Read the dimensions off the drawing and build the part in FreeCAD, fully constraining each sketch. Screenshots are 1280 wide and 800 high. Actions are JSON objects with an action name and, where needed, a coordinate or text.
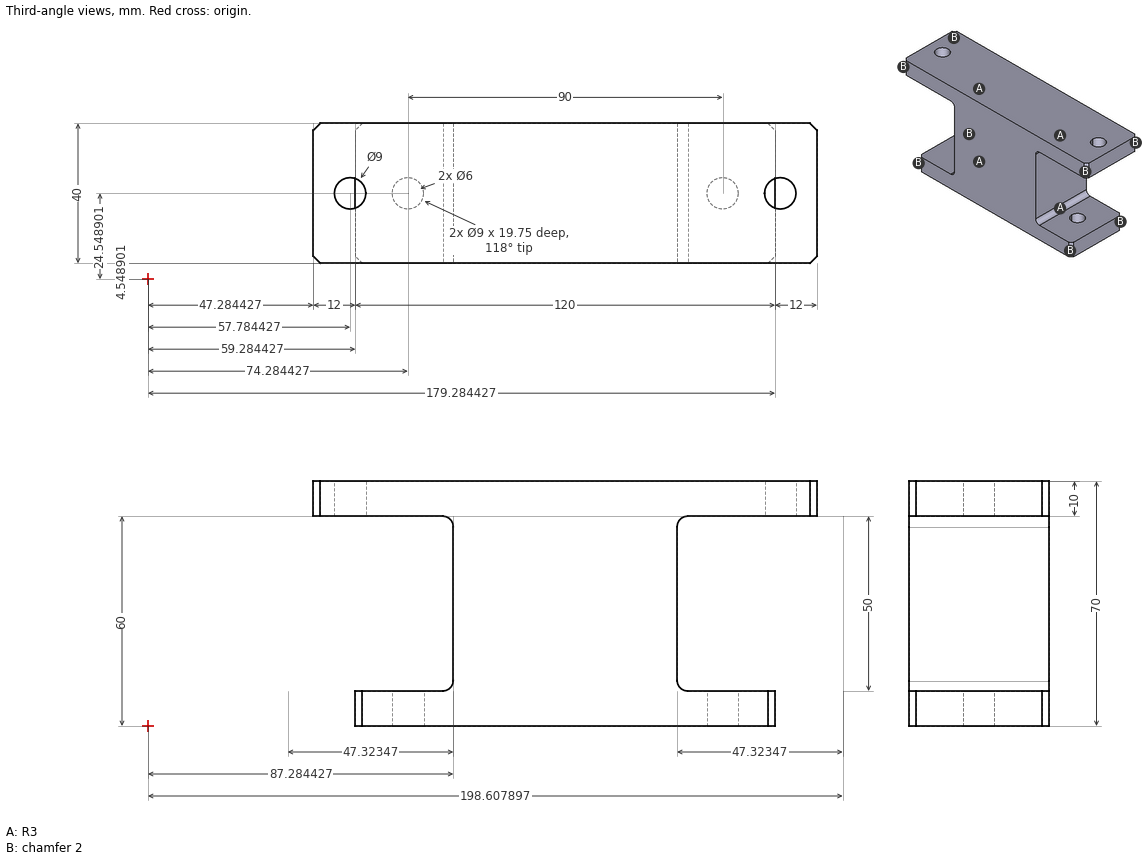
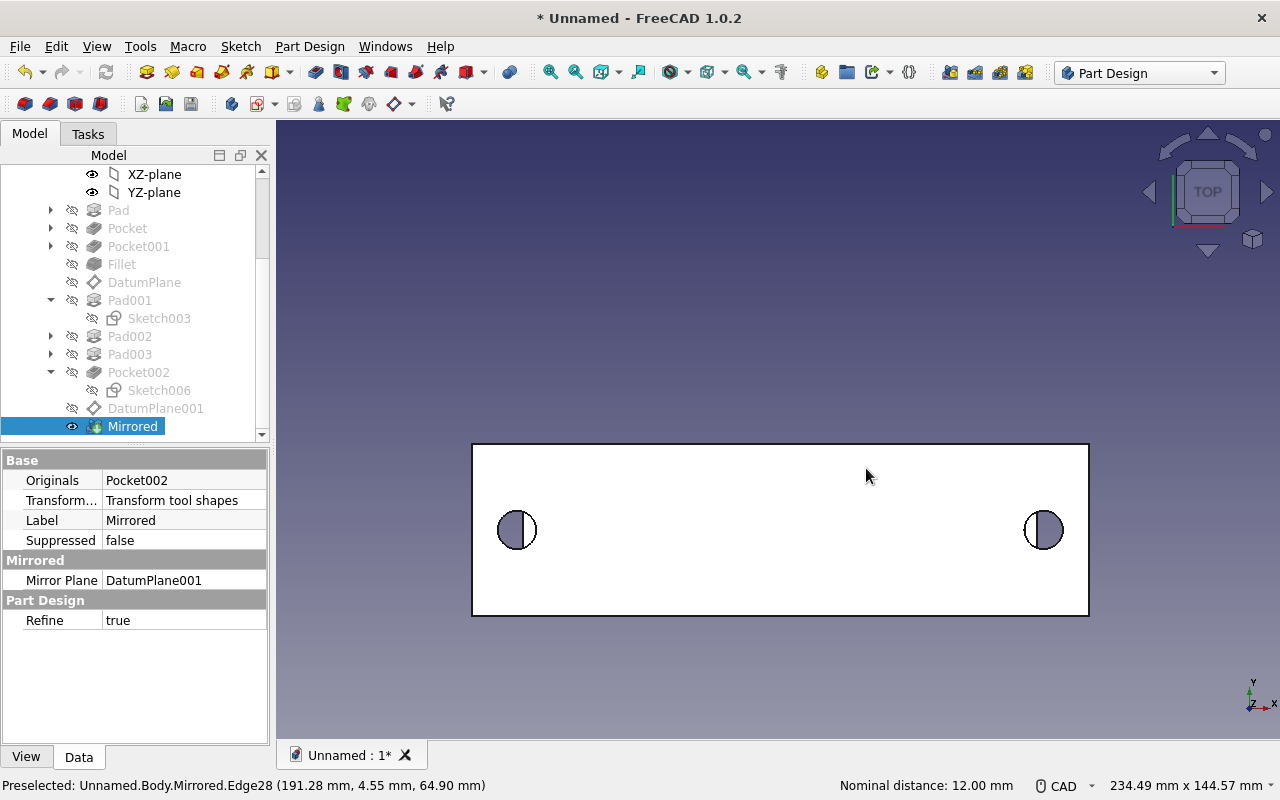
{"action": "key", "text": "0"}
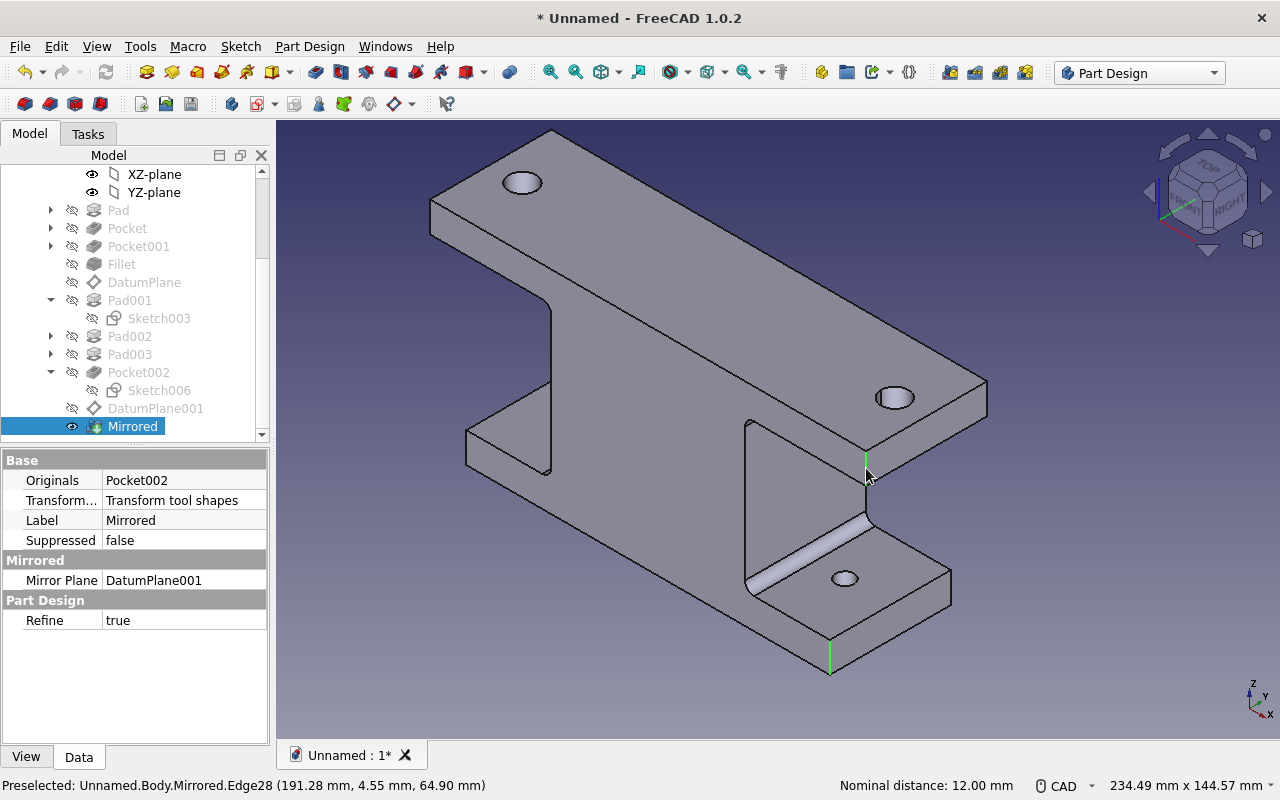
{"action": "key", "text": "1"}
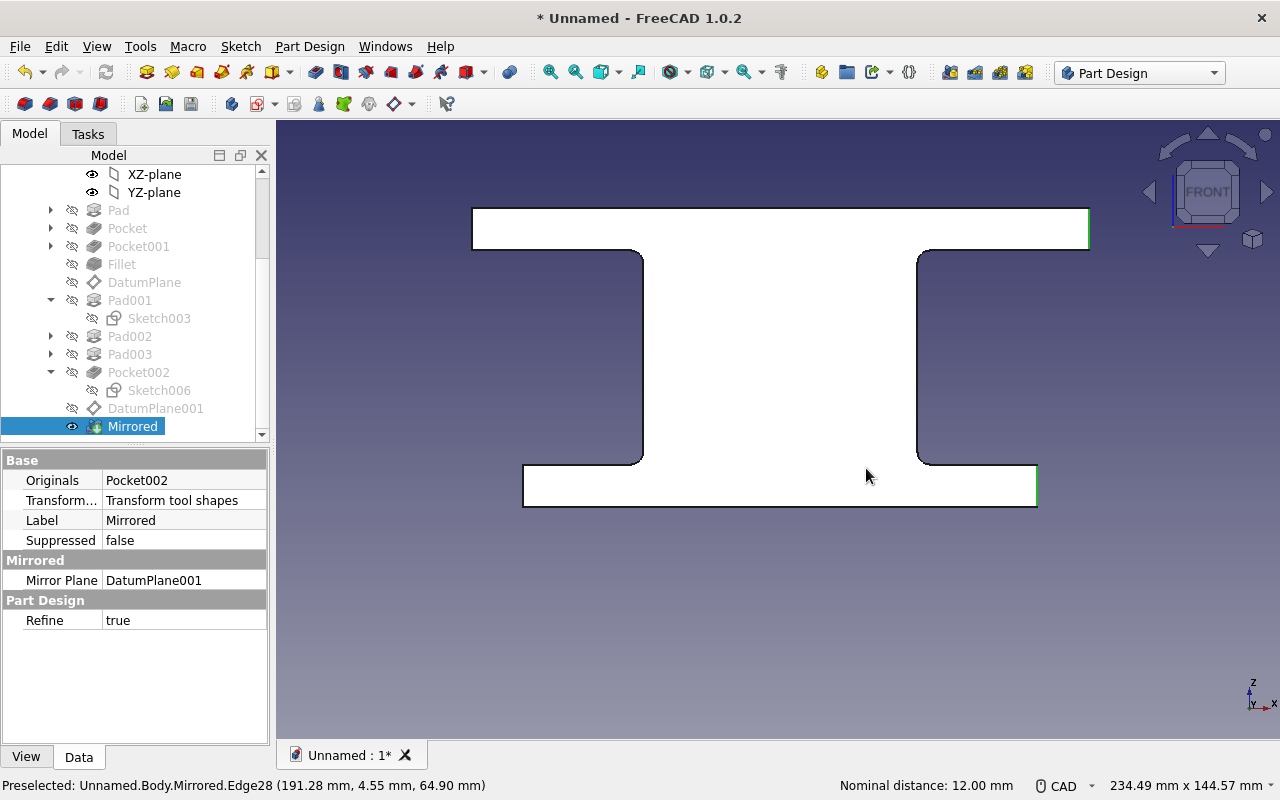
{"action": "left_click", "coordinate": [472, 228], "text": "ctrl"}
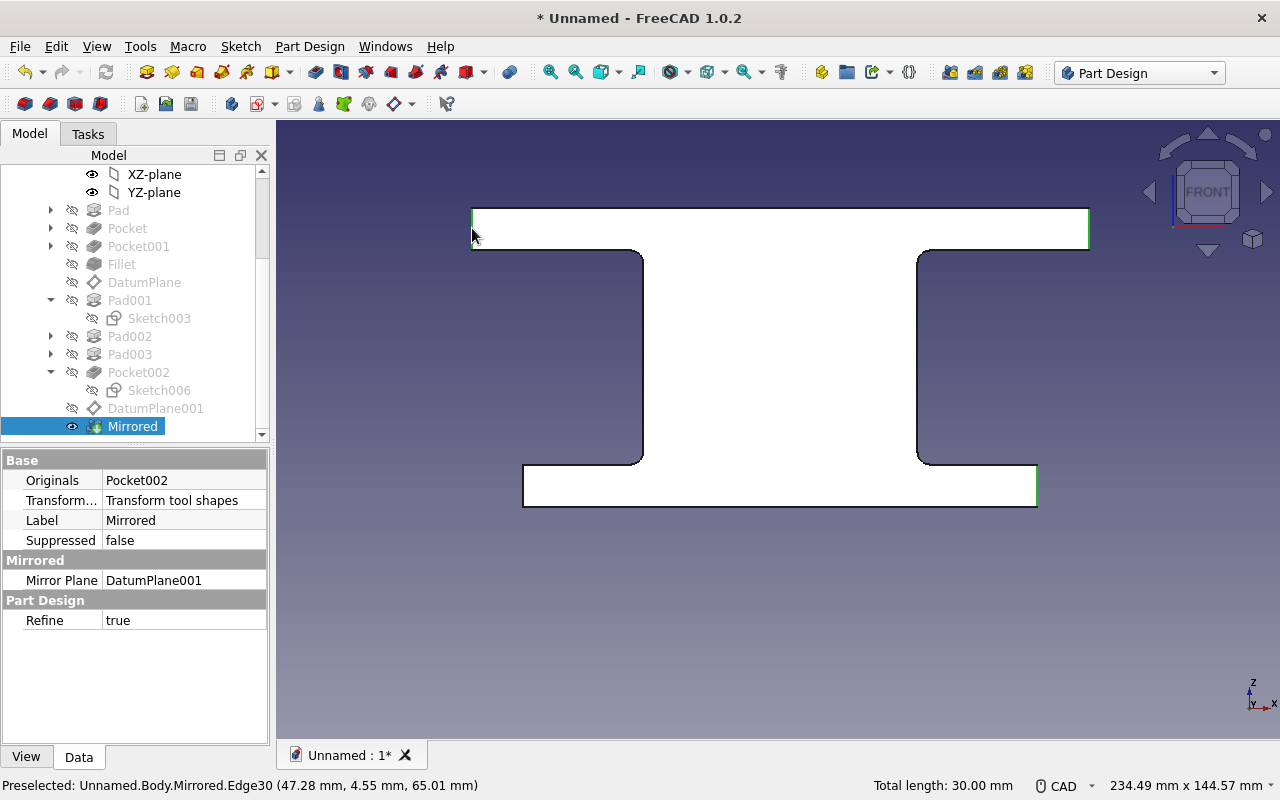
{"action": "left_click", "coordinate": [523, 485], "text": "ctrl"}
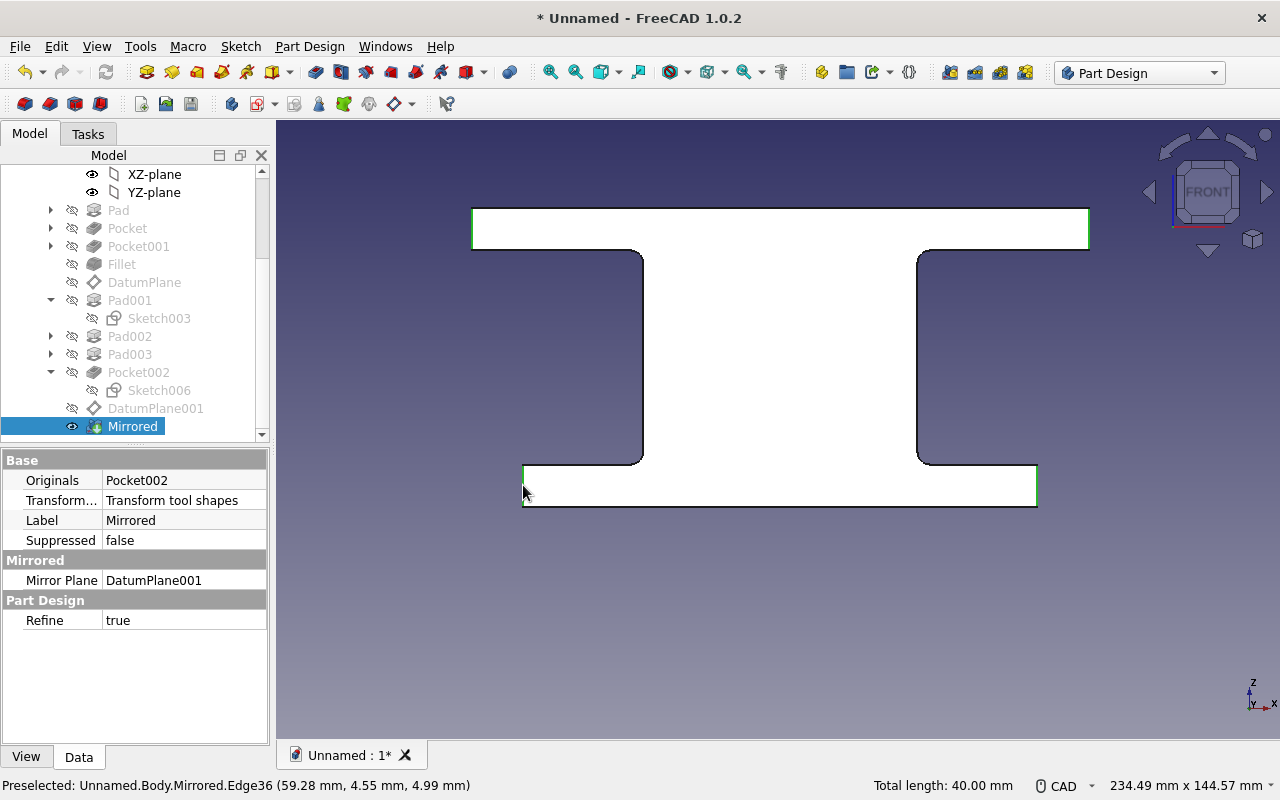
{"action": "key", "text": "3"}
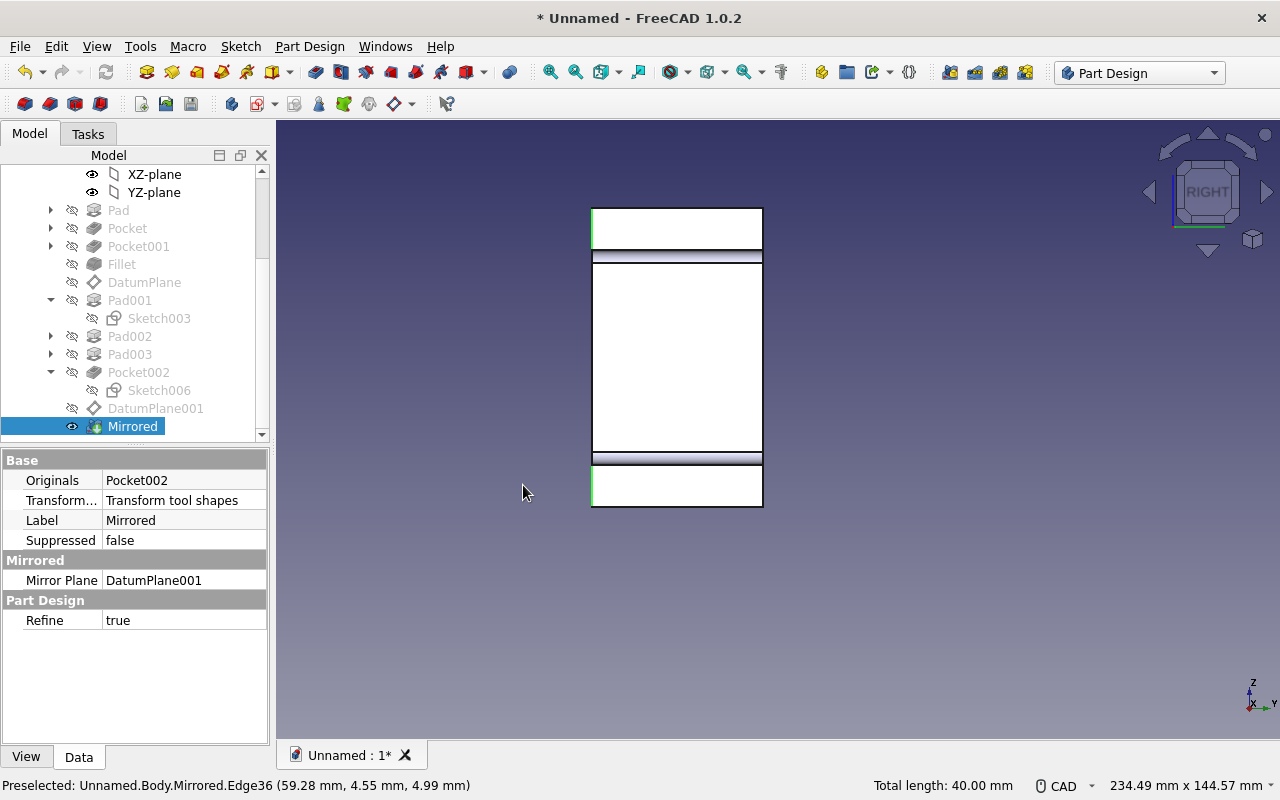
{"action": "left_click", "coordinate": [763, 485], "text": "ctrl"}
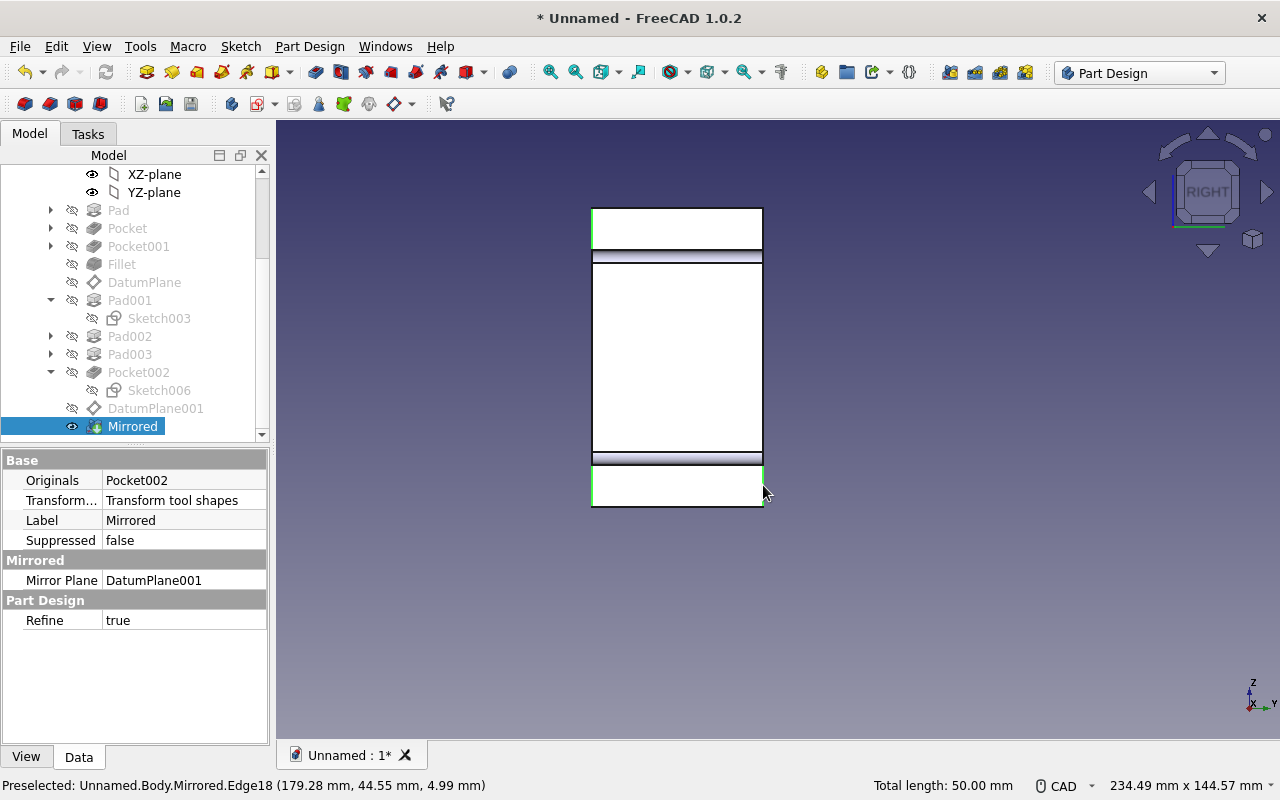
{"action": "left_click", "coordinate": [763, 228], "text": "ctrl"}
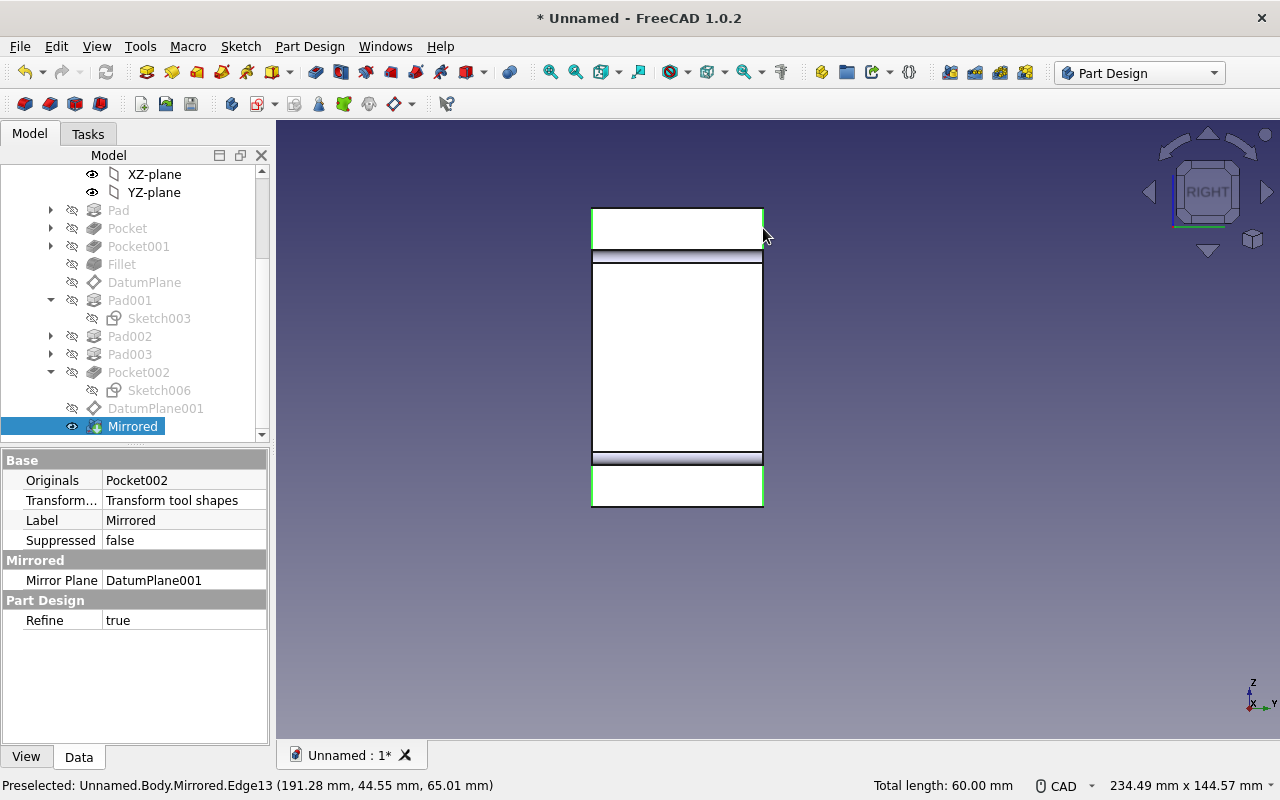
{"action": "key", "text": "5"}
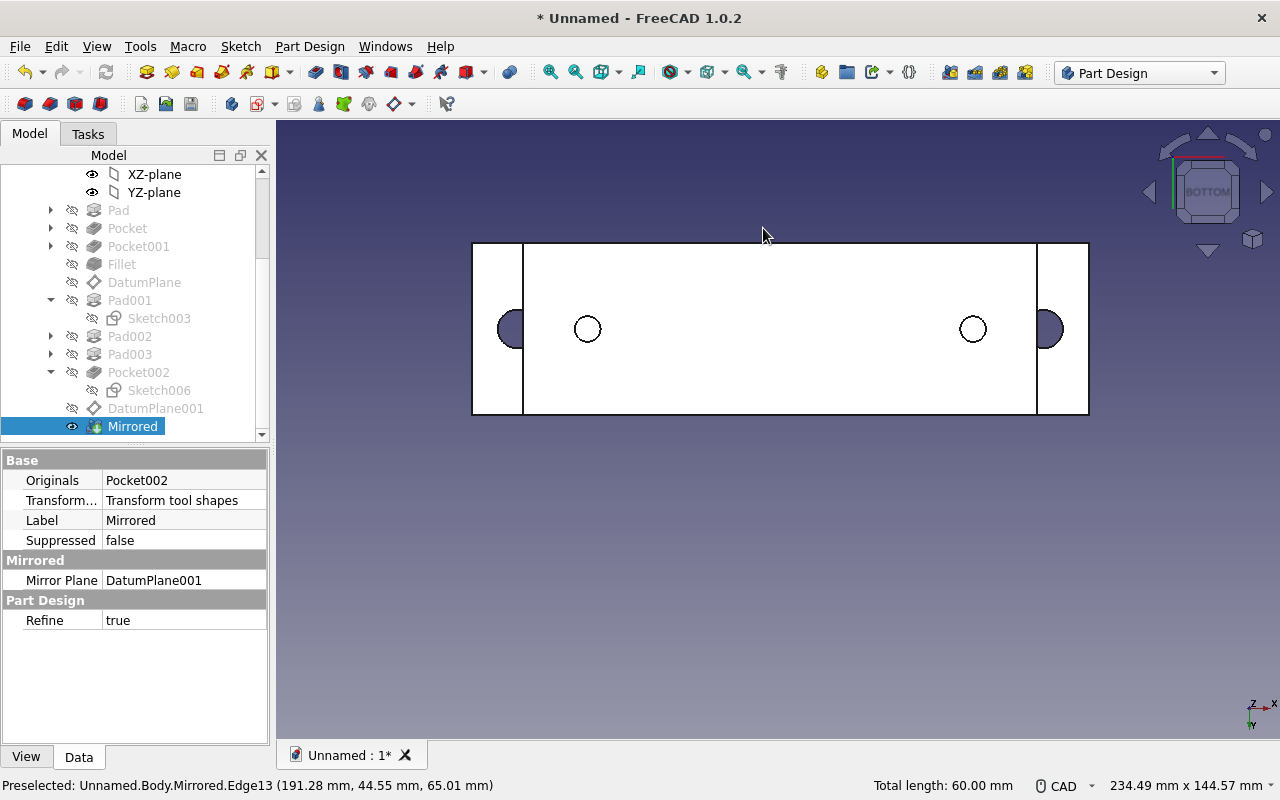
{"action": "key", "text": "4"}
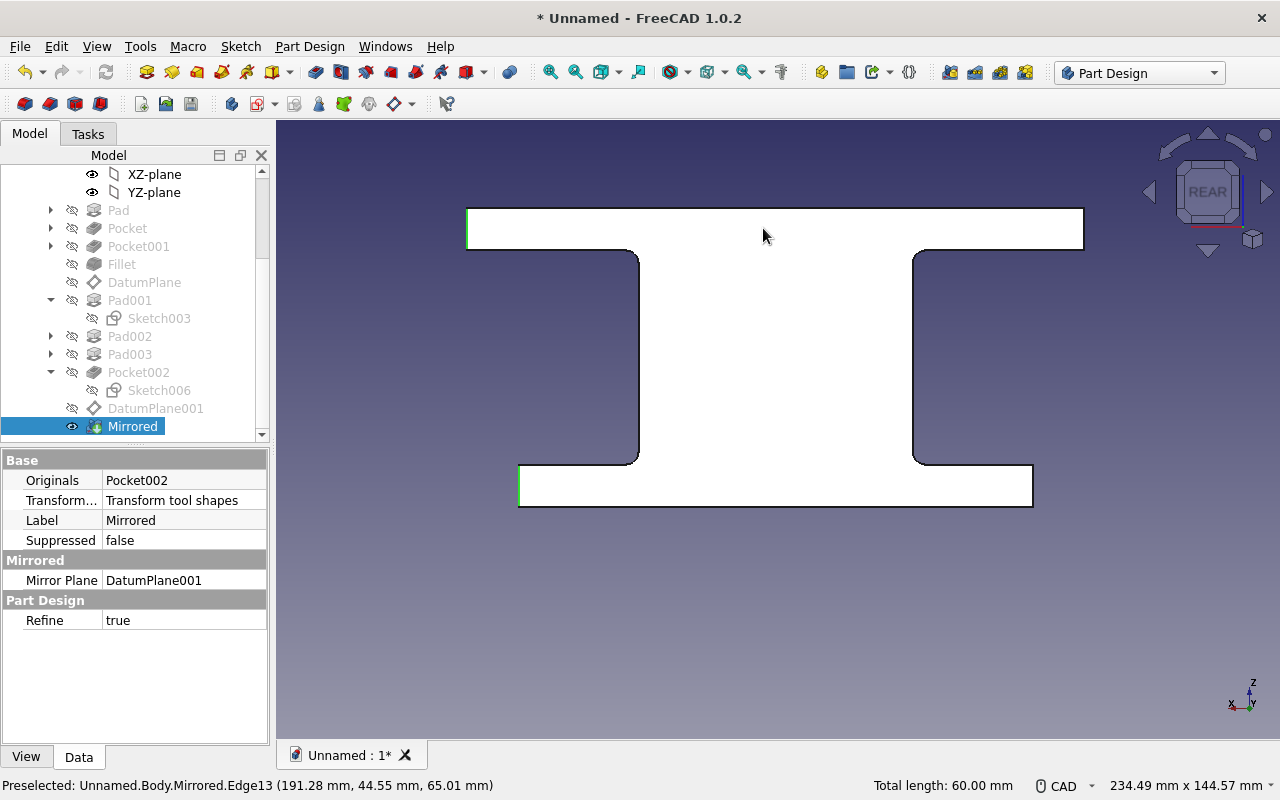
{"action": "left_click", "coordinate": [1084, 228], "text": "ctrl"}